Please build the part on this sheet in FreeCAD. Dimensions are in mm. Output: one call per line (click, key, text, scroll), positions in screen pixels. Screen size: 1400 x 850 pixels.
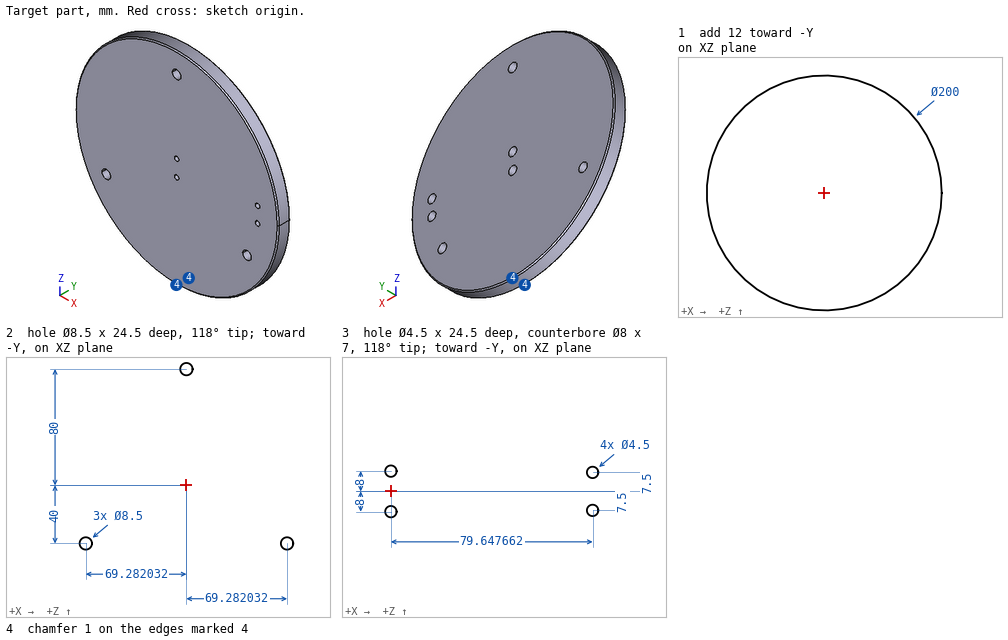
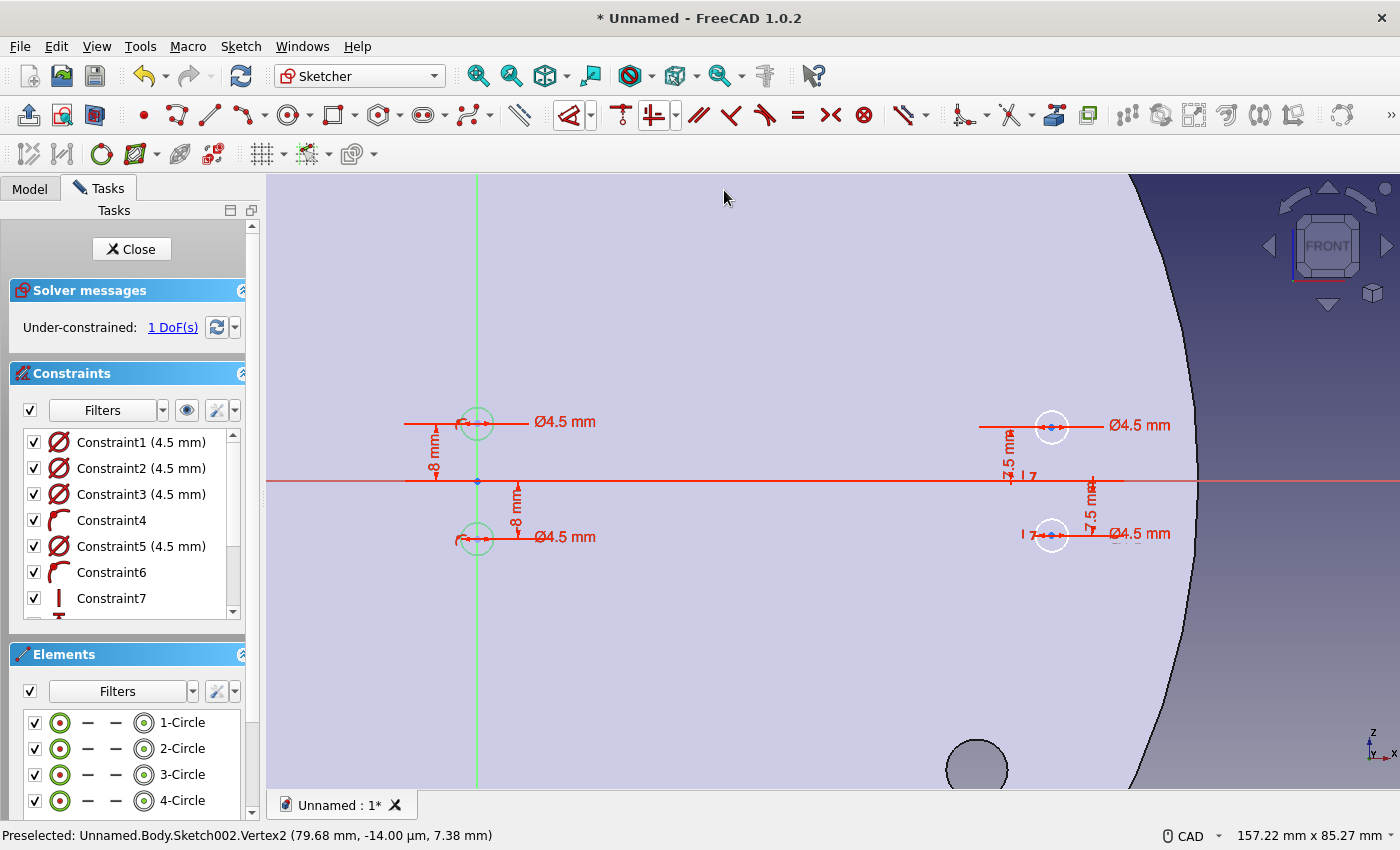
click(1052, 536)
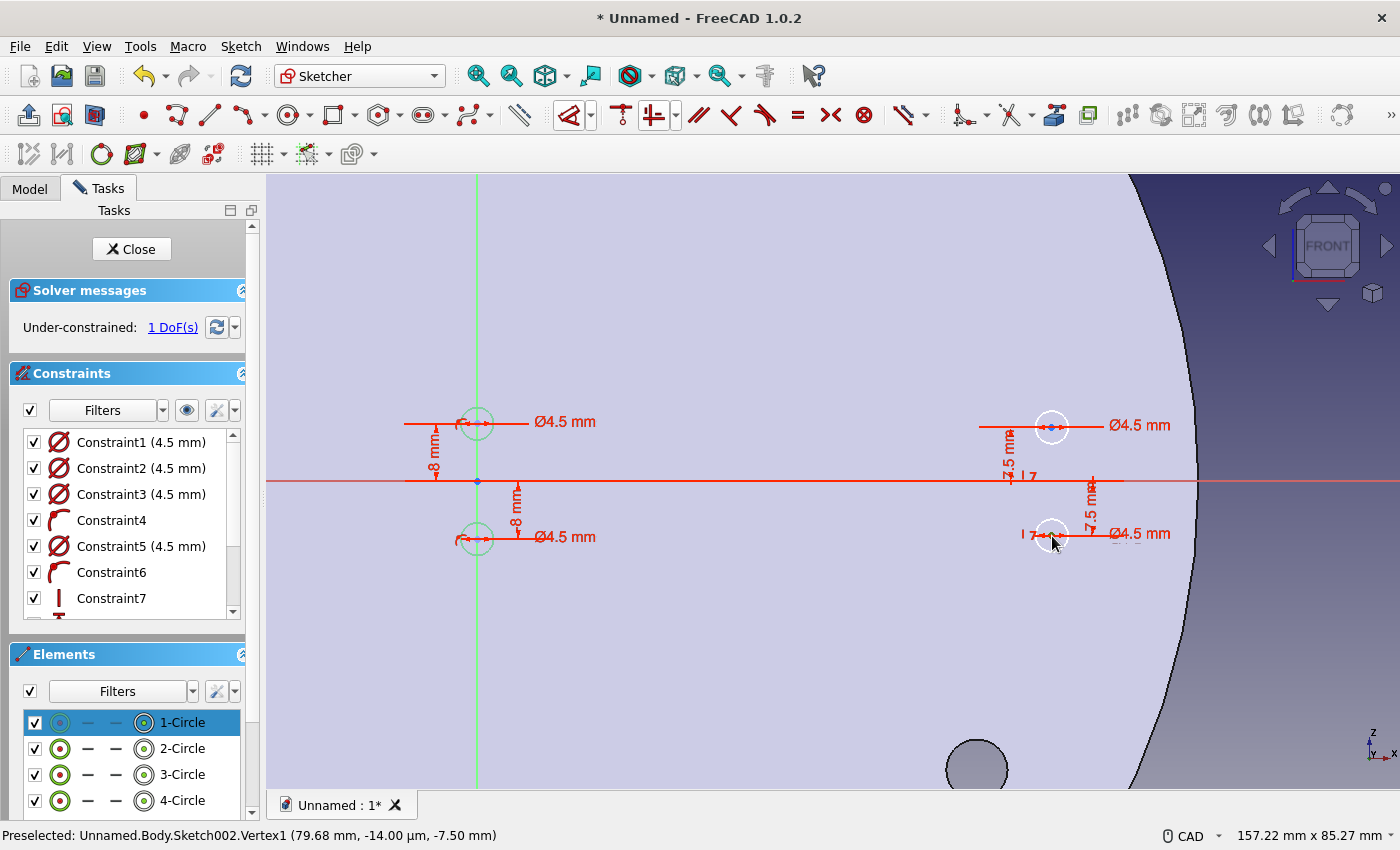
key(l)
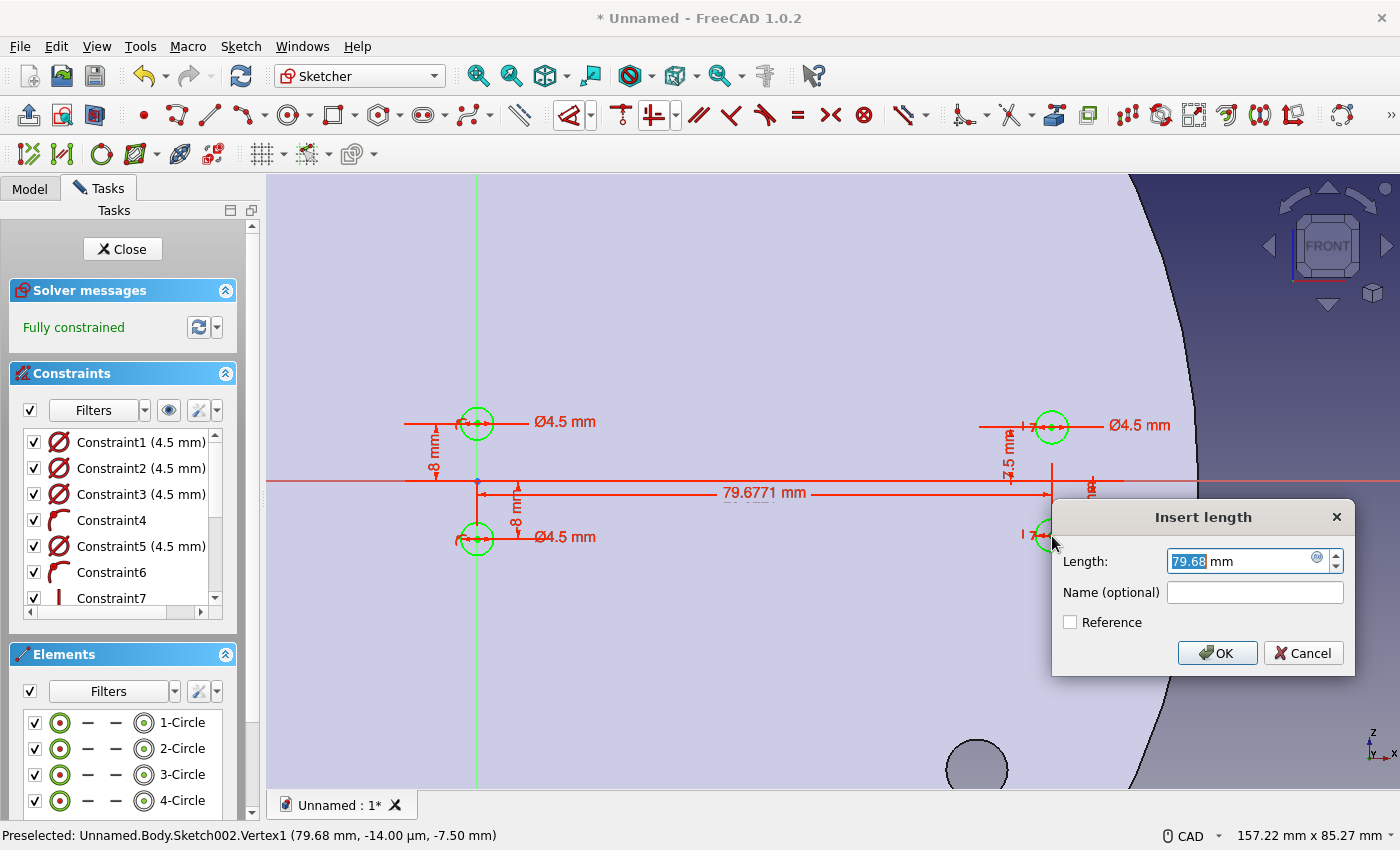
text(79.647662)
key(Return)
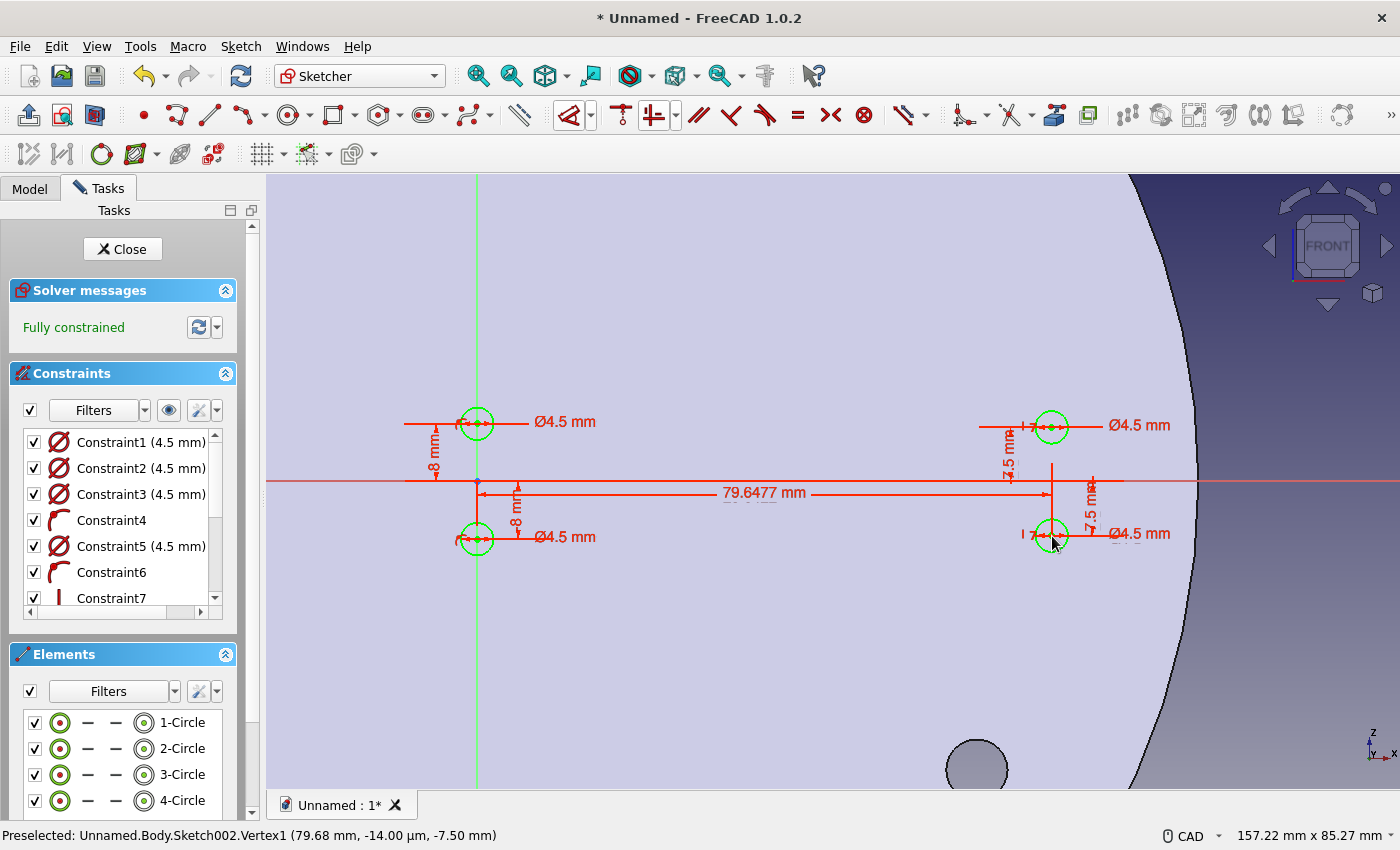
click(123, 249)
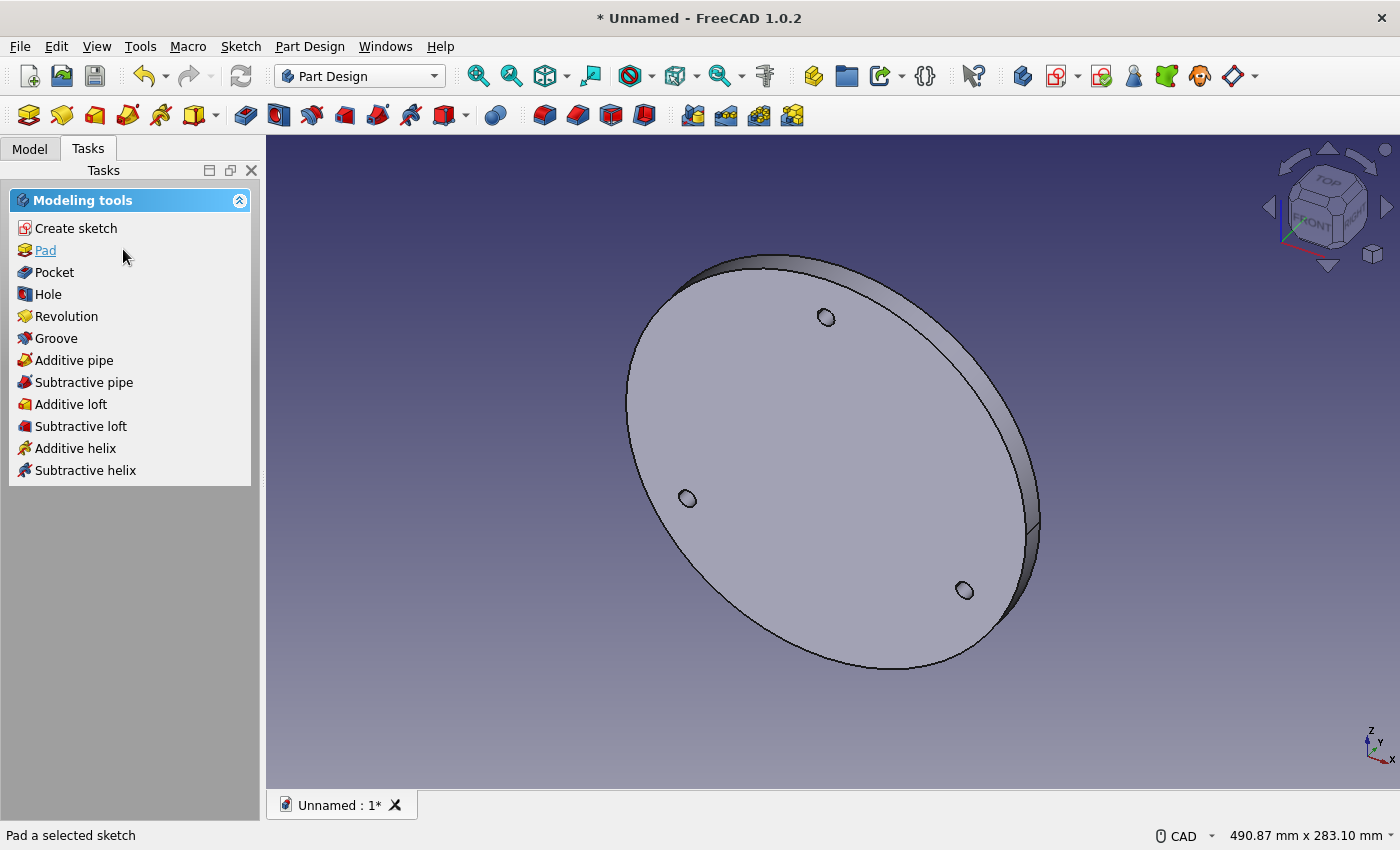
click(279, 116)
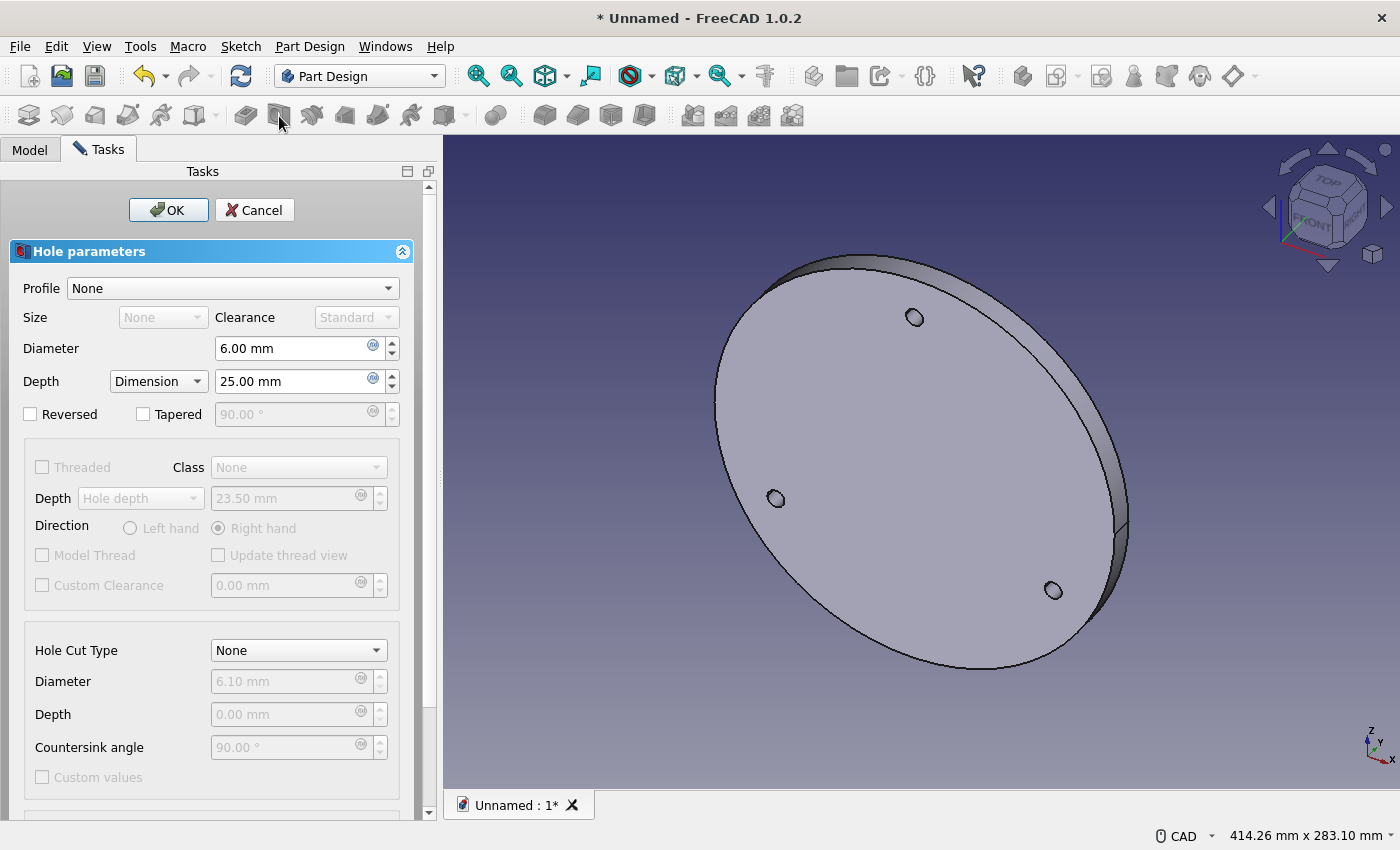
triple_click(300, 348)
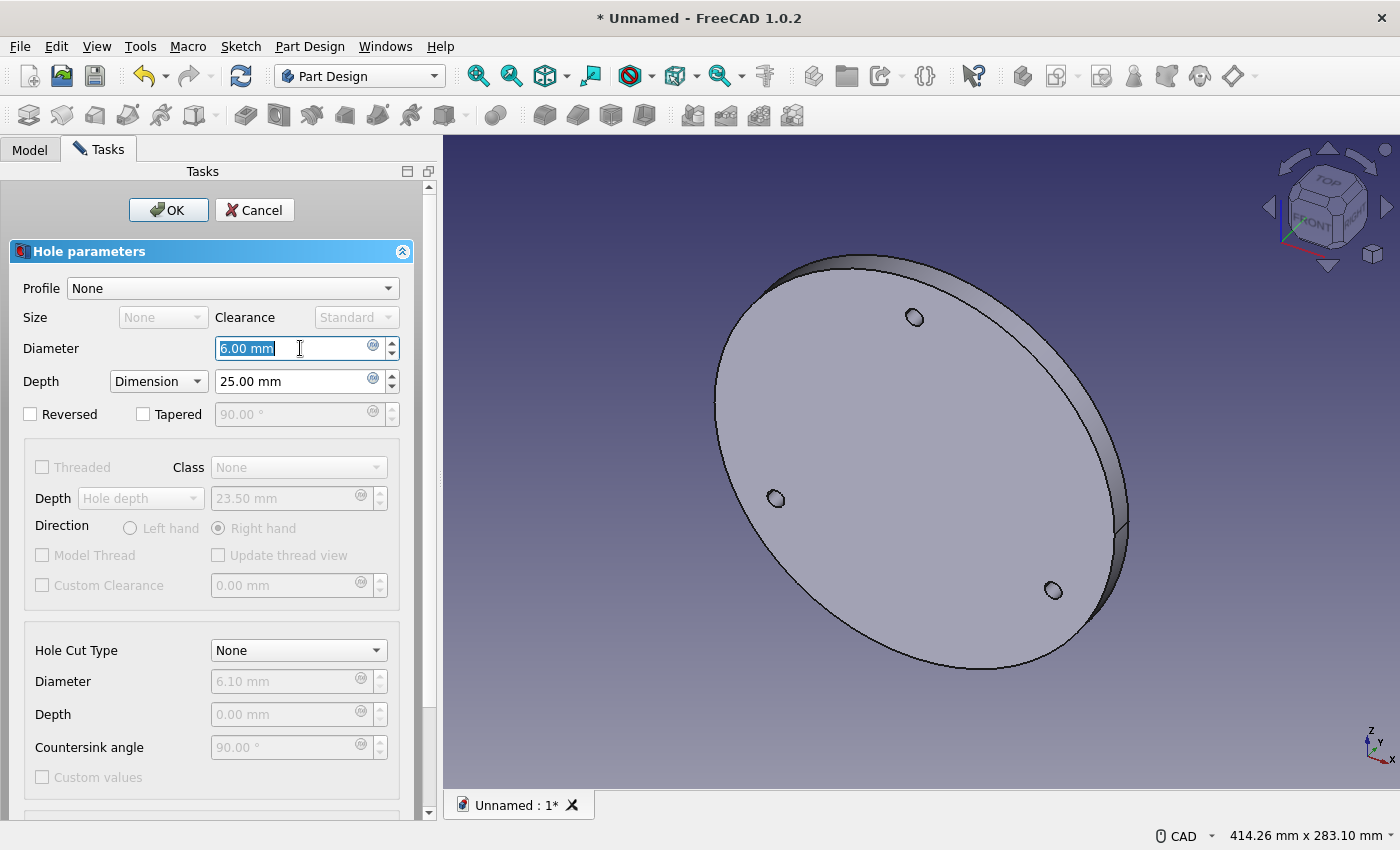
text(4.5)
key(Tab)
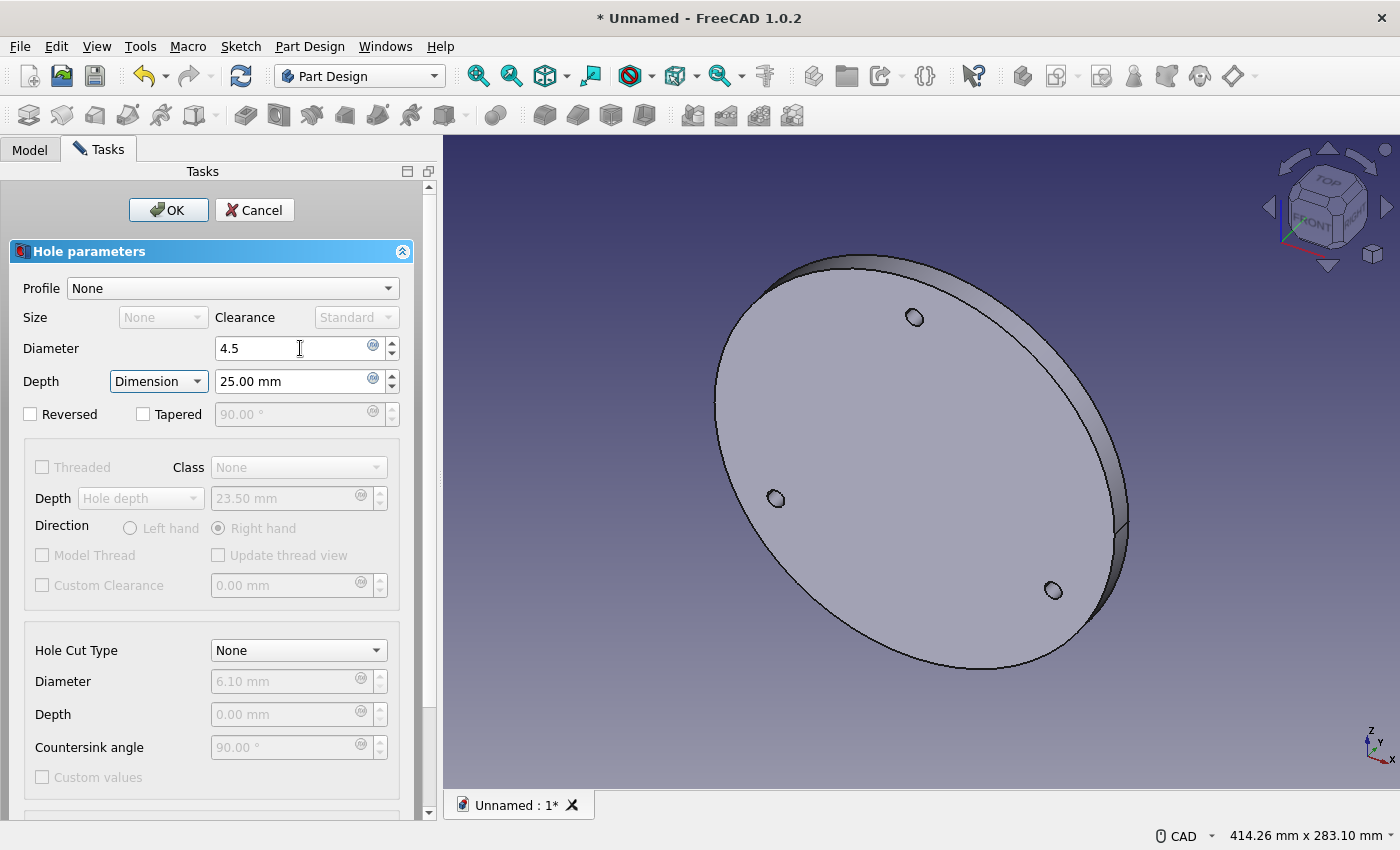
triple_click(300, 382)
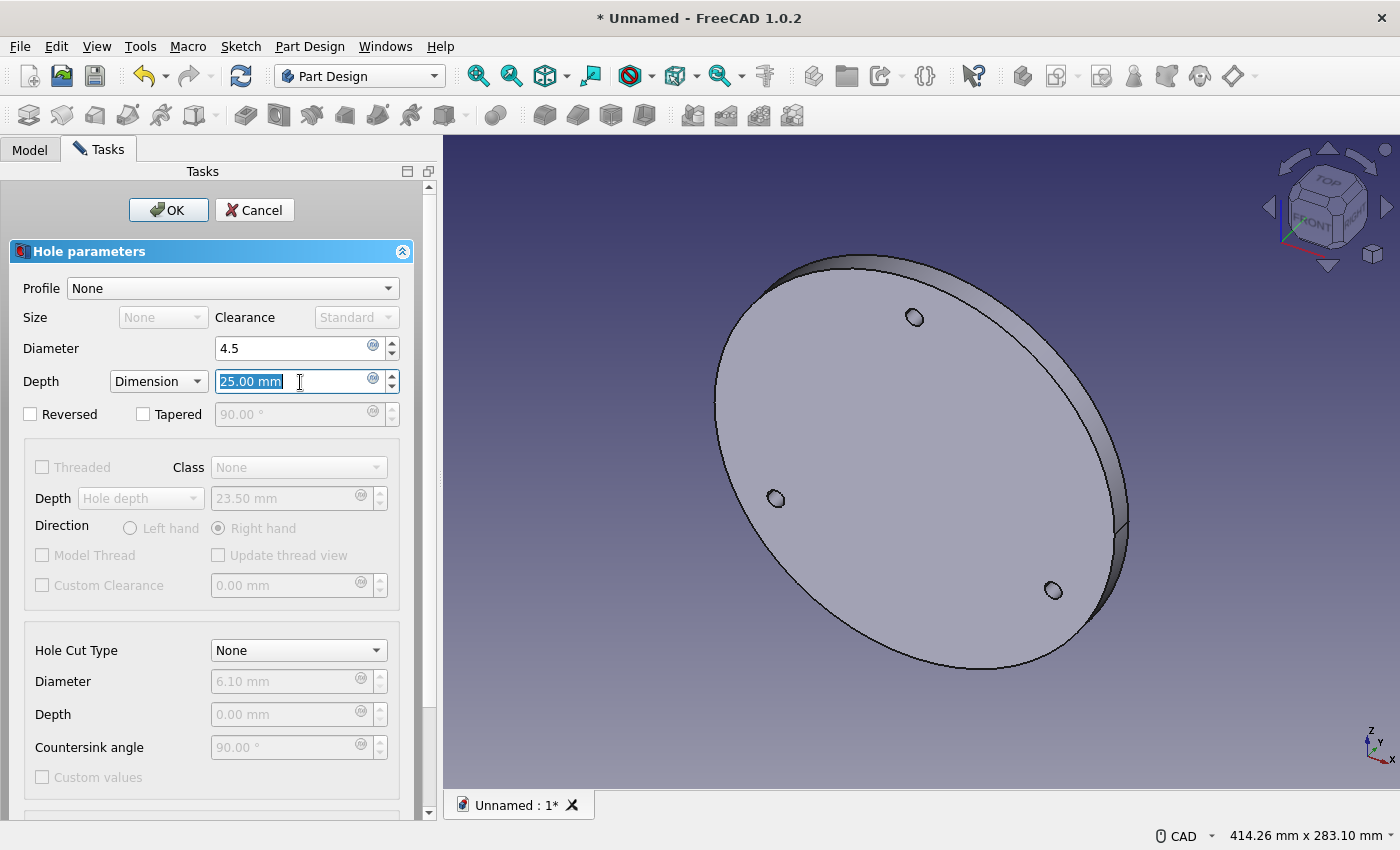
text(24.5)
key(Tab)